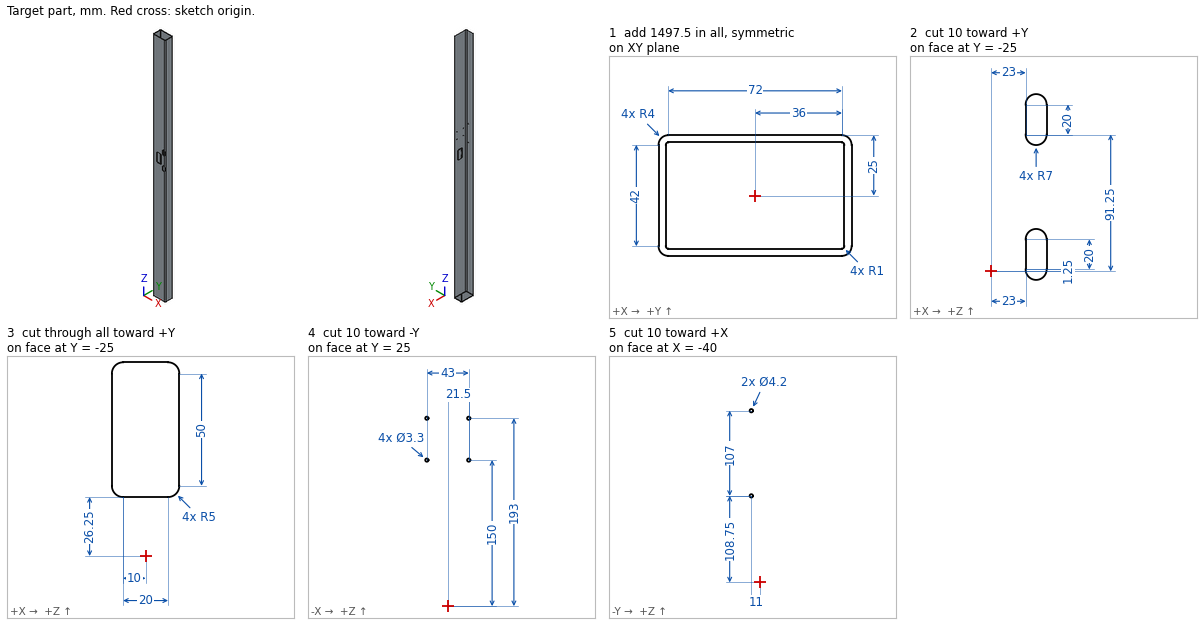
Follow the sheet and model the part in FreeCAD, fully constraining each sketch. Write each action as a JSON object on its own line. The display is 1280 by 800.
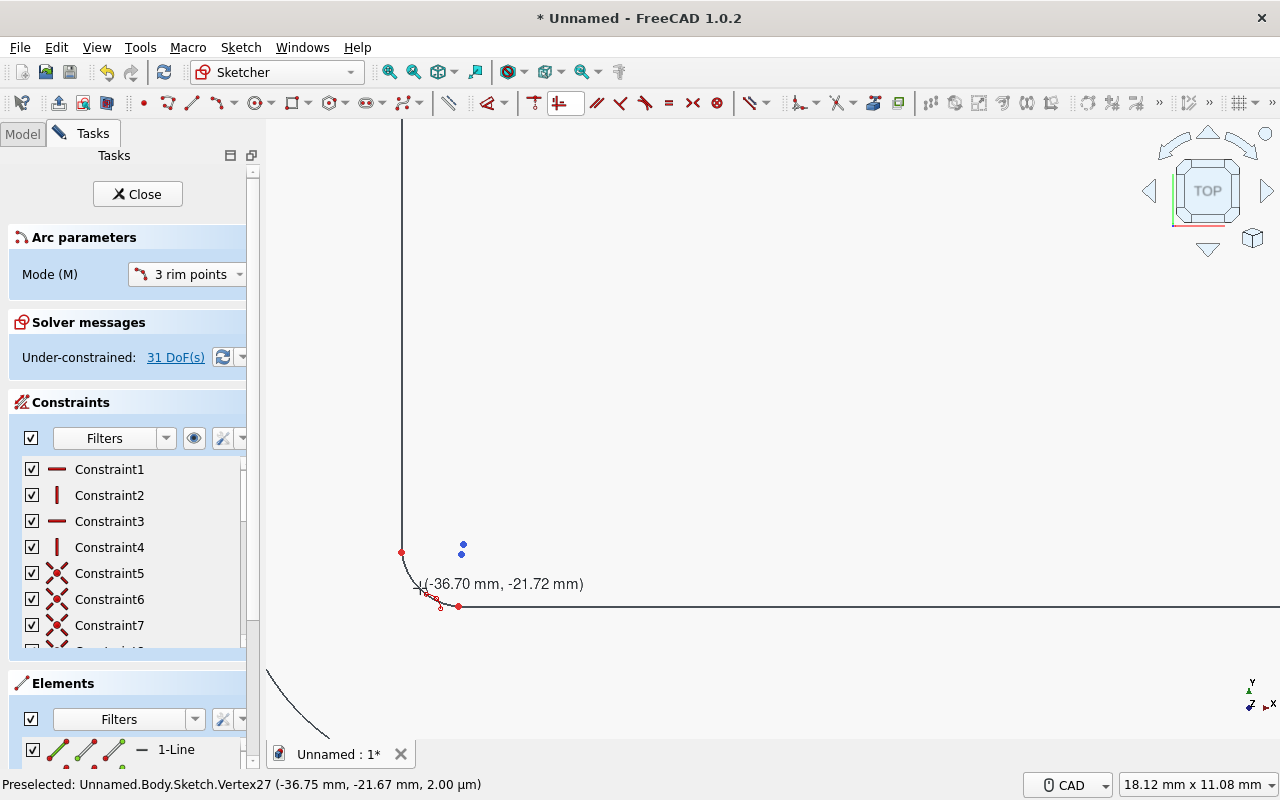
{"action": "scroll", "coordinate": [428, 594], "scroll_direction": "down", "scroll_amount": 10}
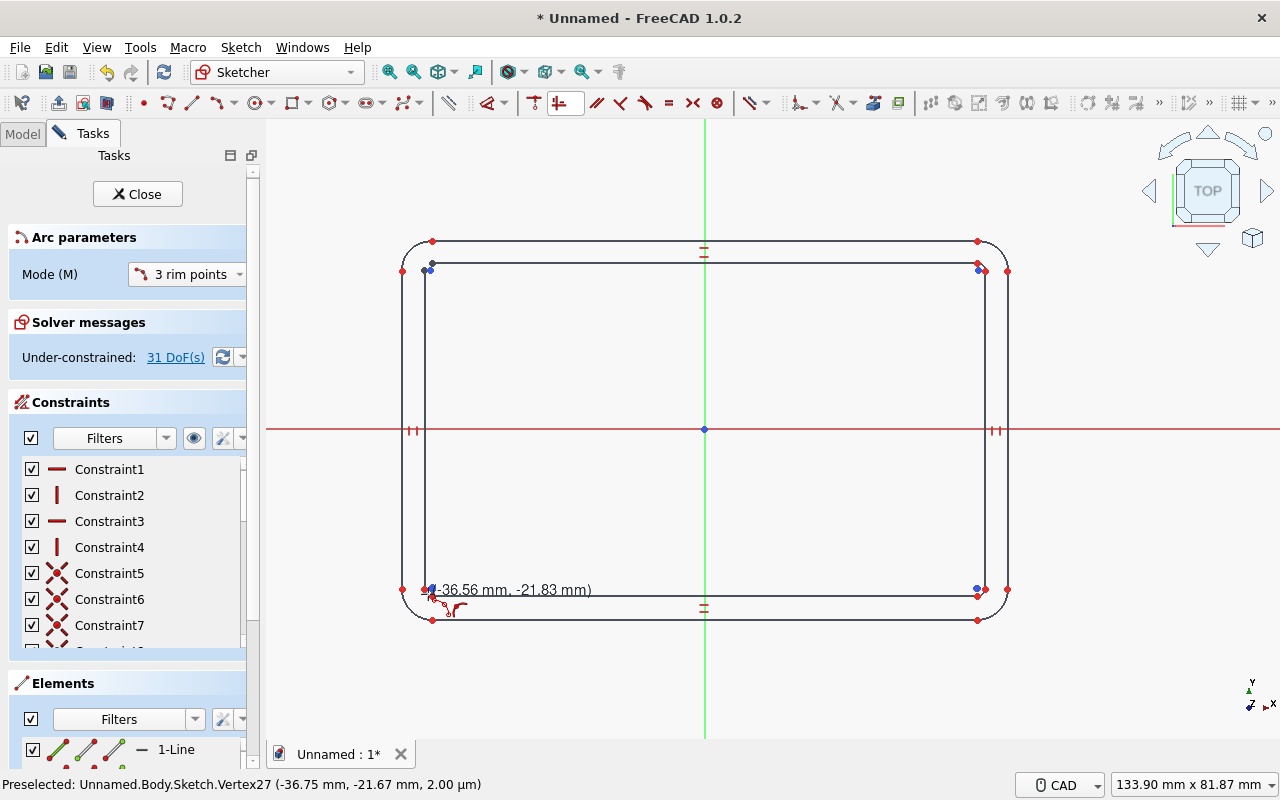
{"action": "scroll", "coordinate": [425, 270], "scroll_direction": "up", "scroll_amount": 4}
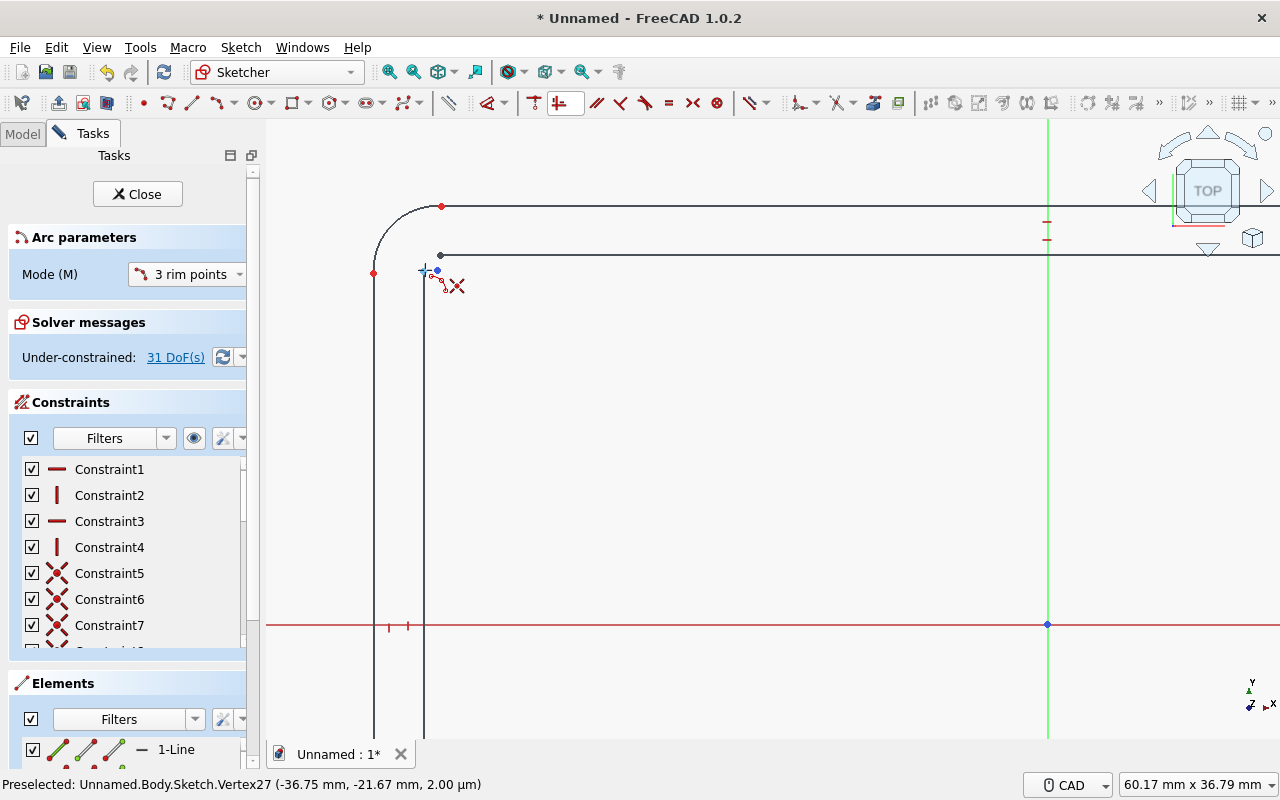
{"action": "left_click", "coordinate": [424, 272]}
{"action": "left_click", "coordinate": [441, 255]}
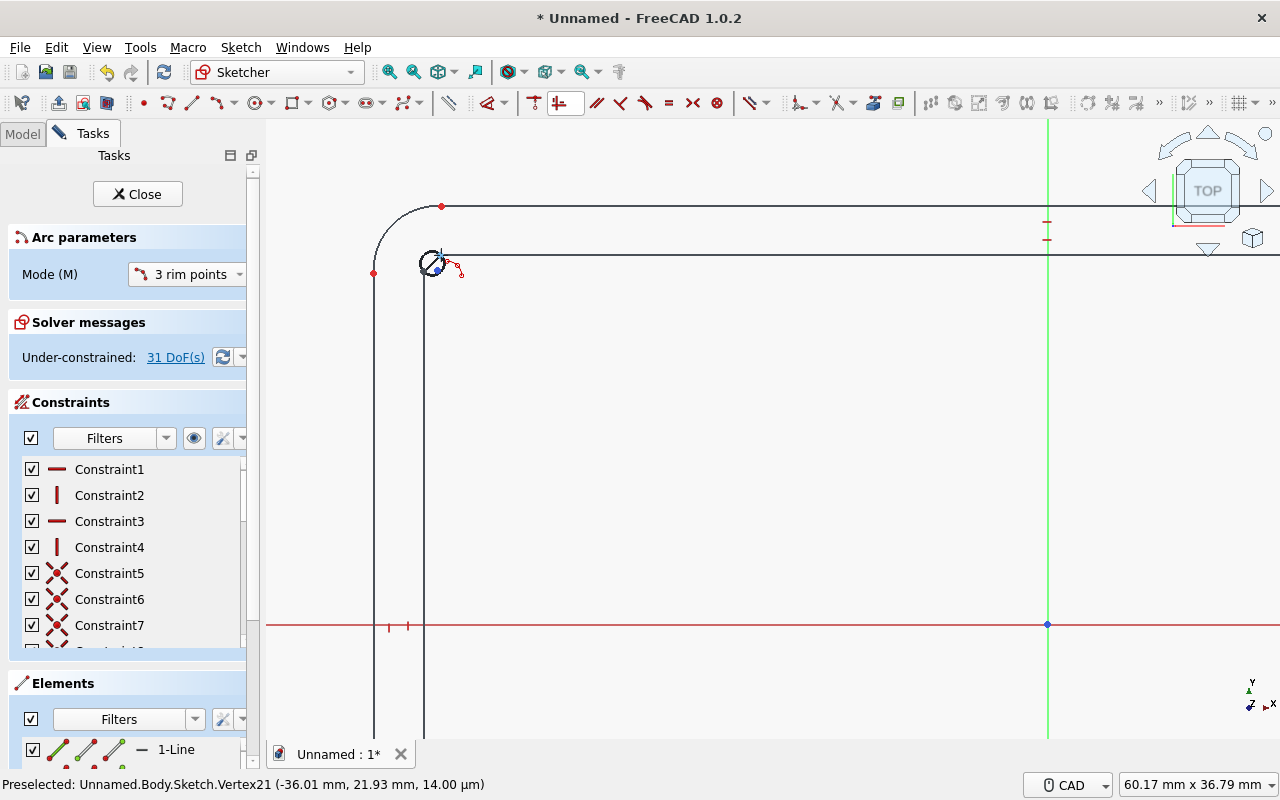
{"action": "scroll", "coordinate": [429, 259], "scroll_direction": "up", "scroll_amount": 6}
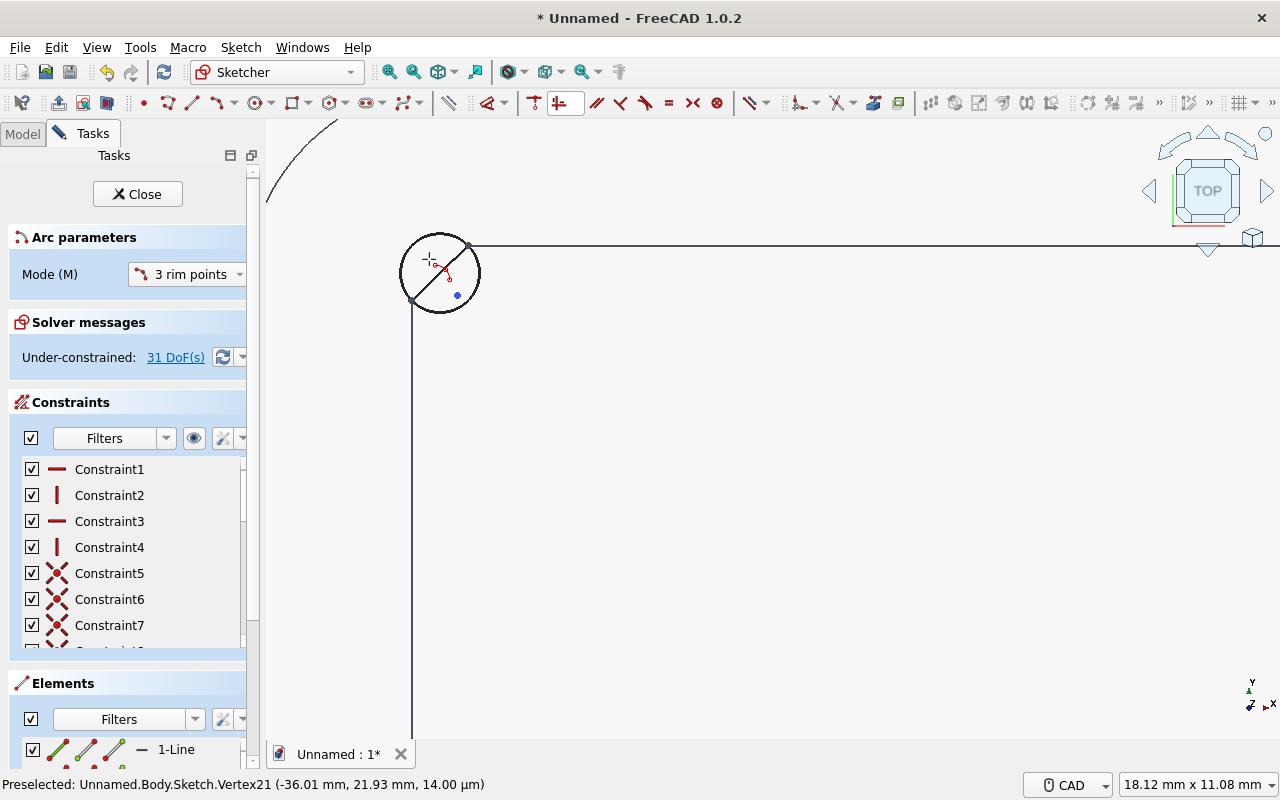
{"action": "left_click", "coordinate": [429, 258]}
{"action": "key", "text": "Escape"}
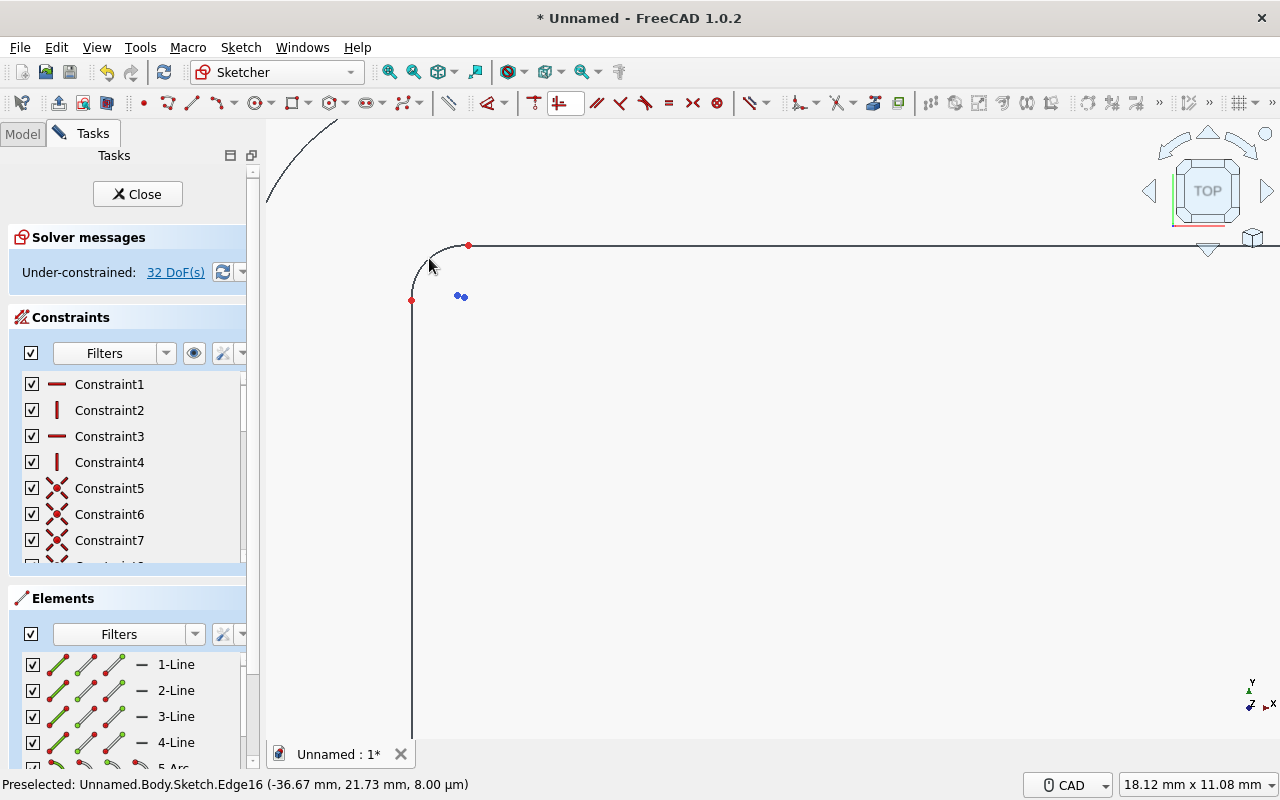
{"action": "scroll", "coordinate": [426, 266], "scroll_direction": "down", "scroll_amount": 10}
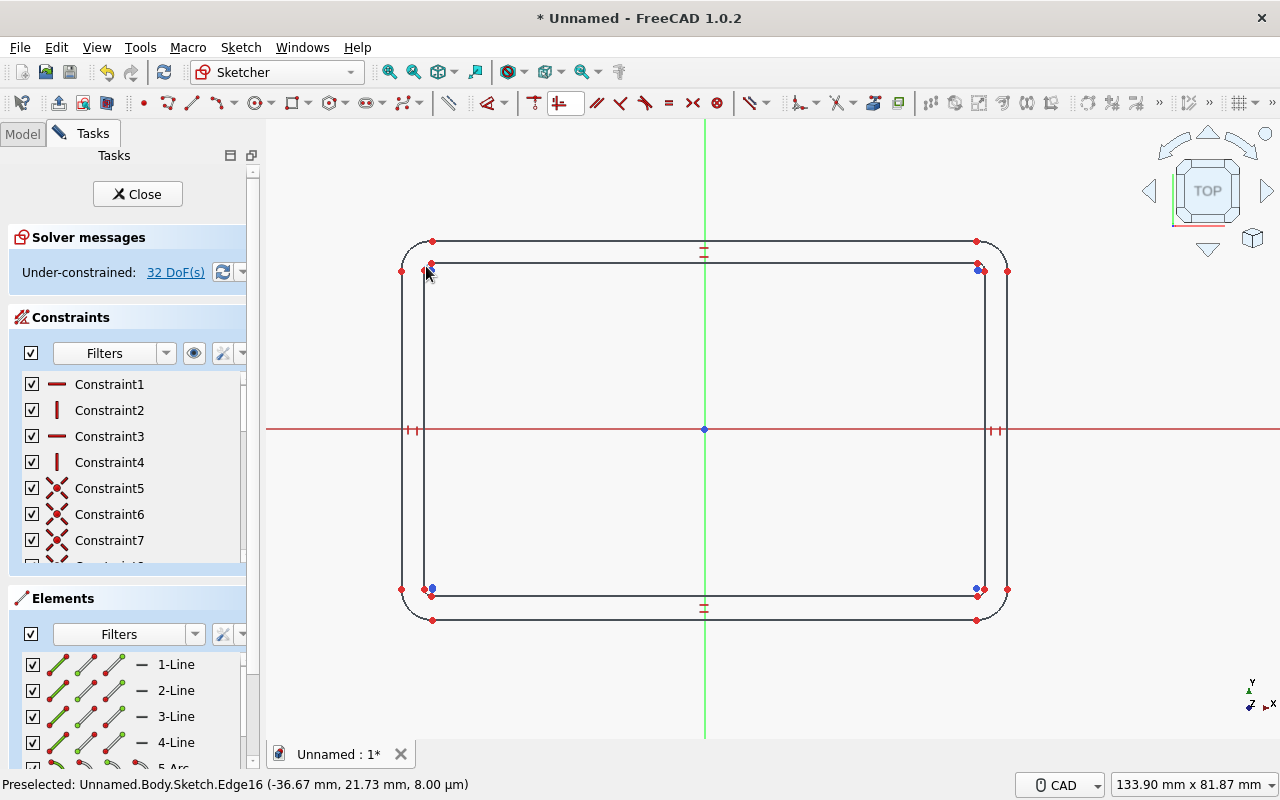
{"action": "left_click", "coordinate": [814, 241]}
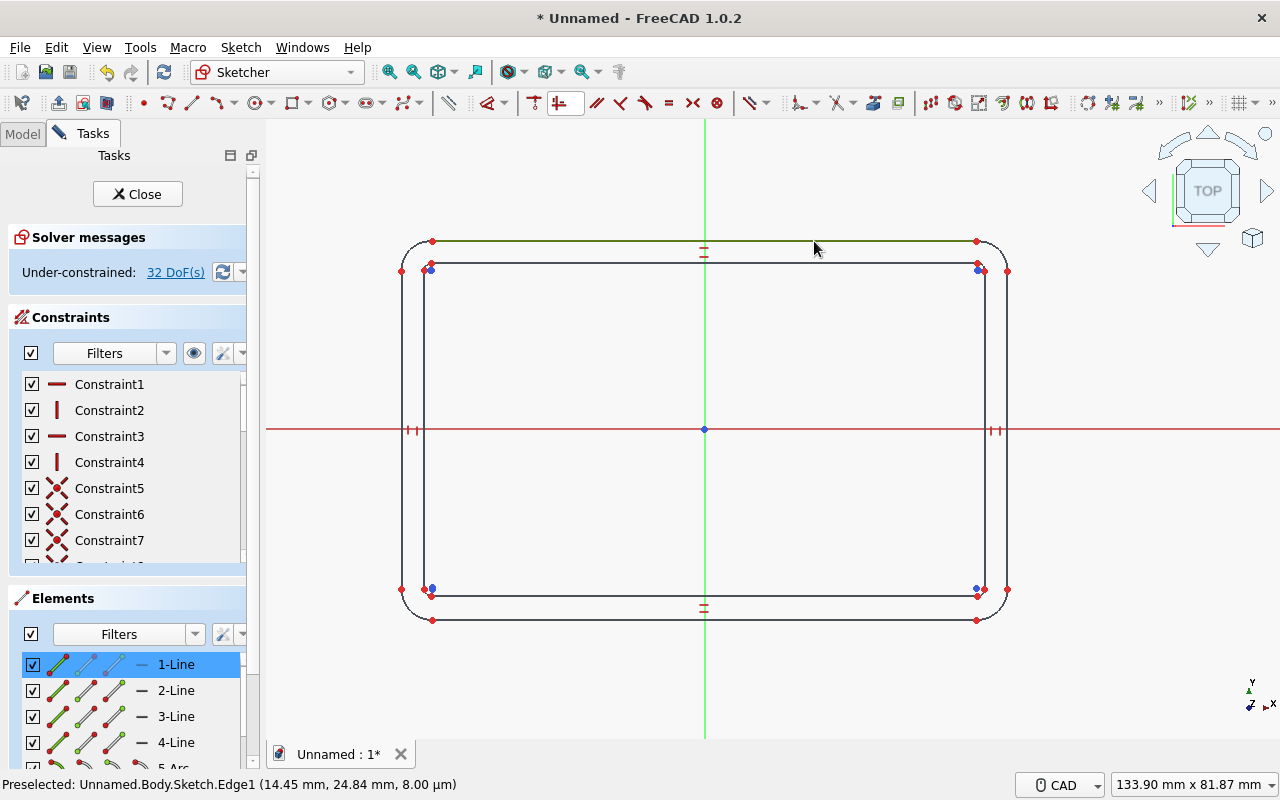
{"action": "left_click", "coordinate": [418, 244]}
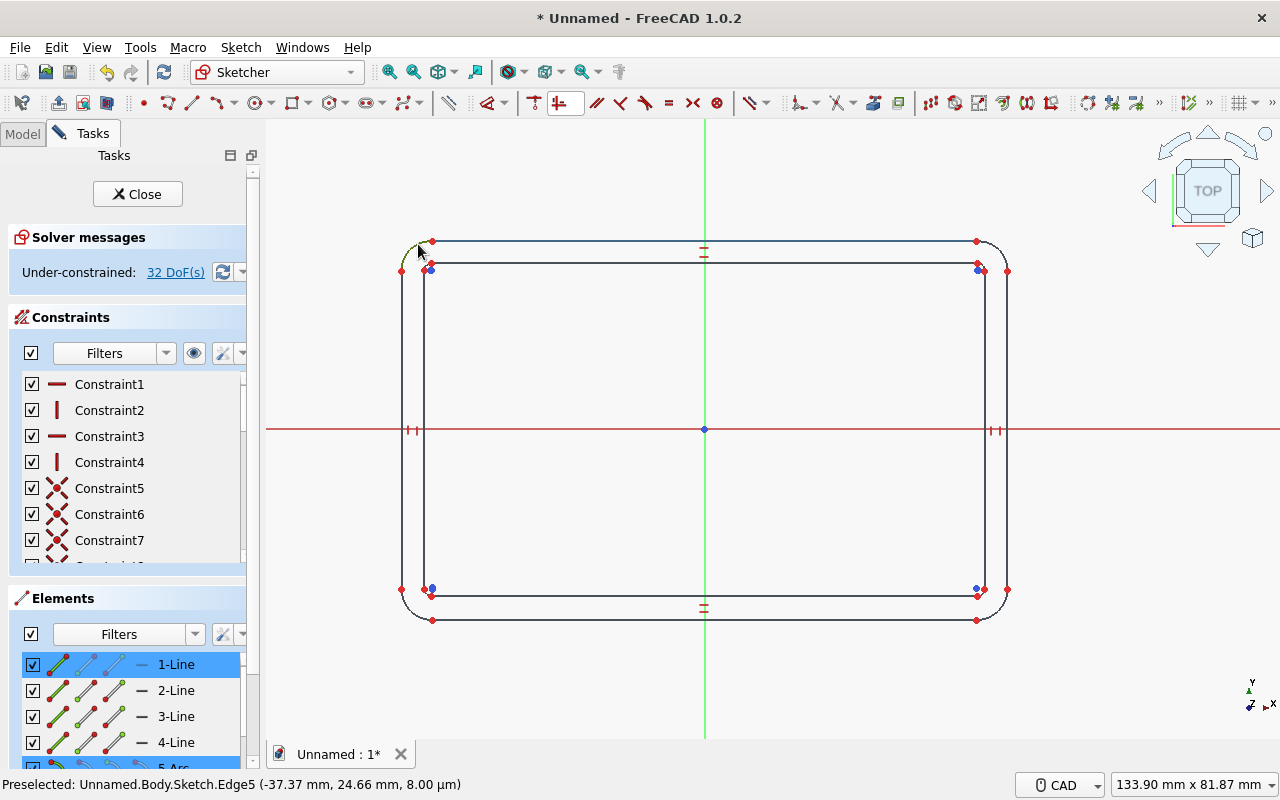
{"action": "left_click", "coordinate": [646, 104]}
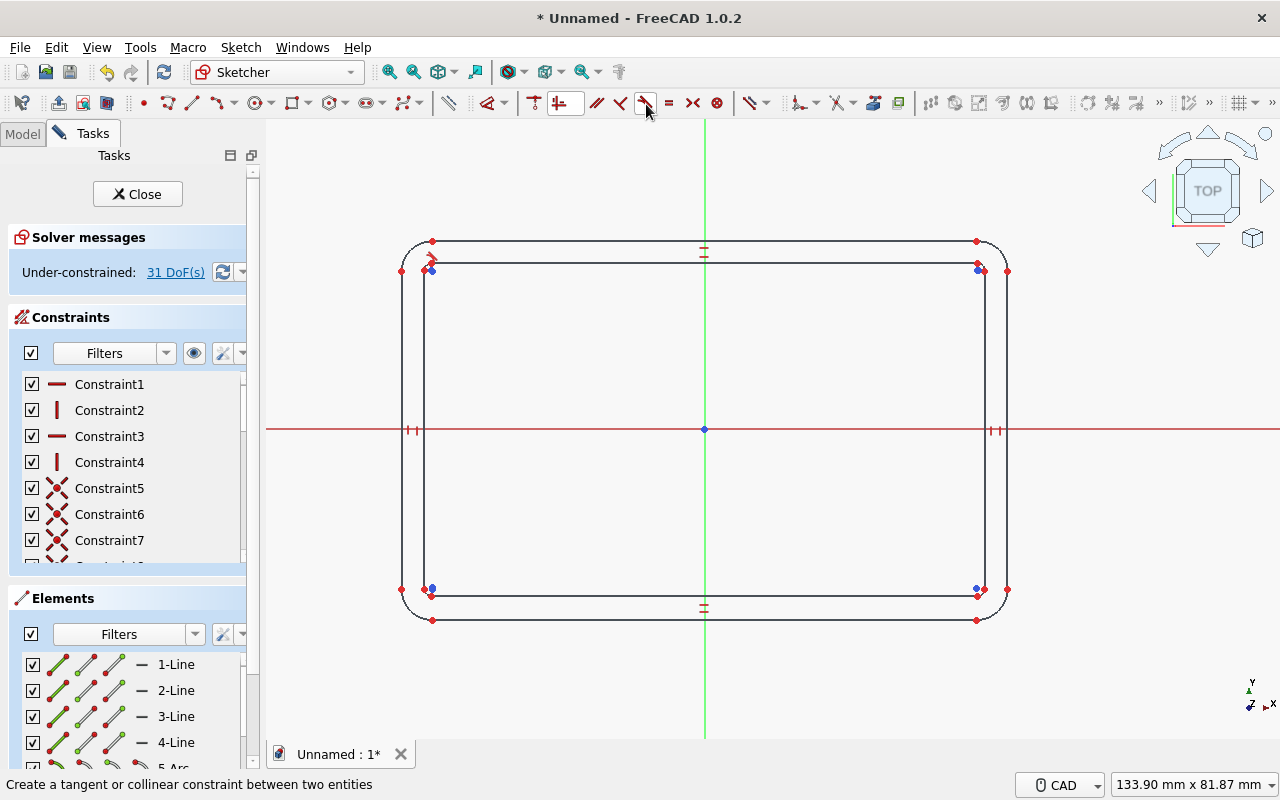
{"action": "left_click", "coordinate": [814, 241]}